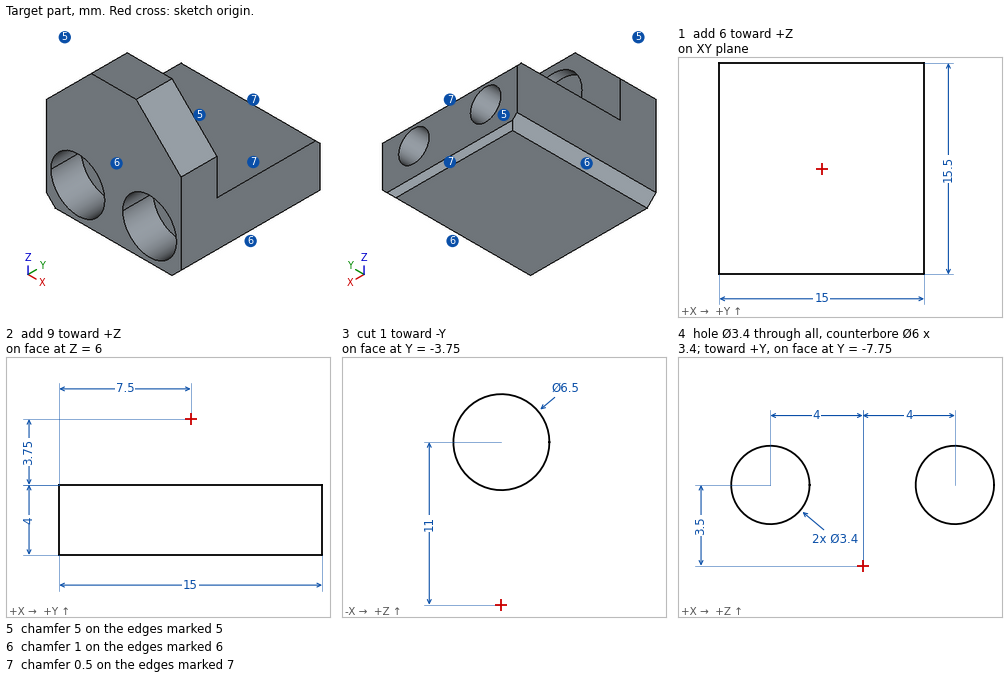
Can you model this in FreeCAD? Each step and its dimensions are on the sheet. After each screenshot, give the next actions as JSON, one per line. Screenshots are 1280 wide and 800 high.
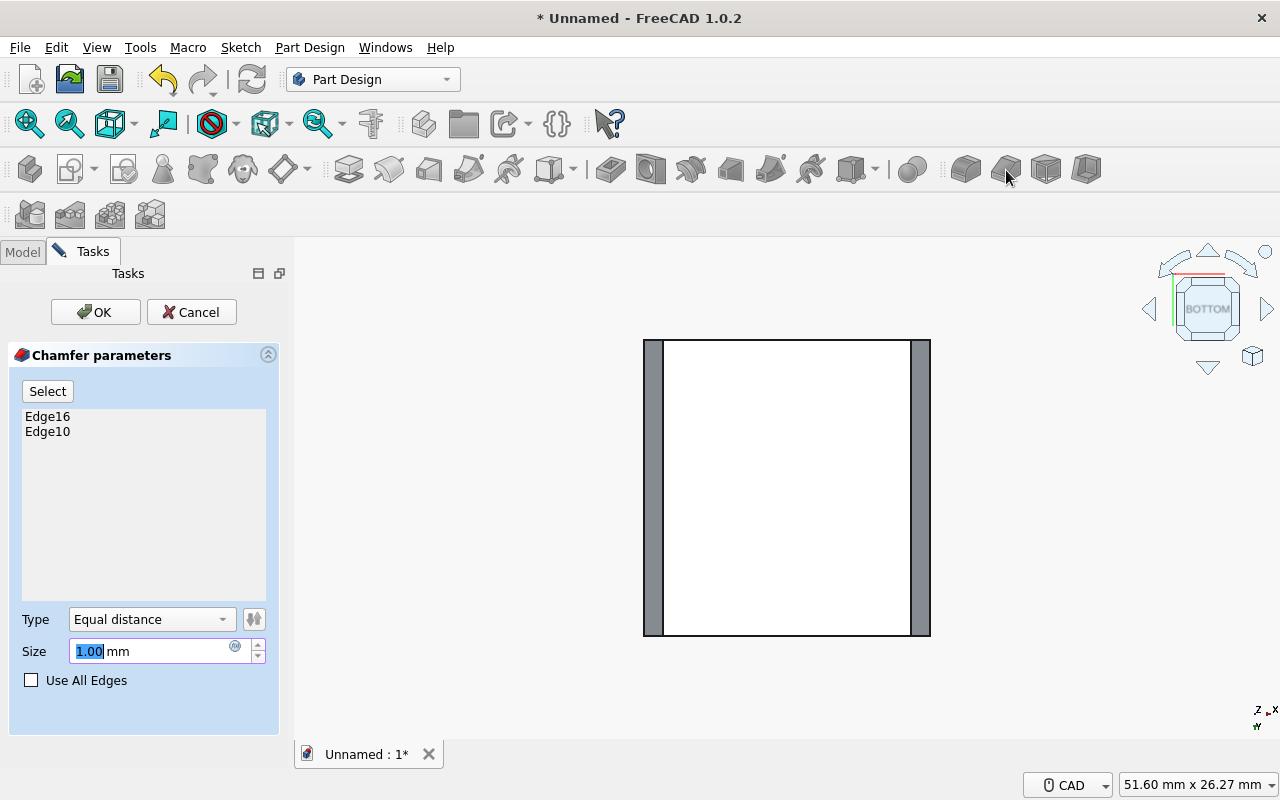
{"action": "type", "text": "1"}
{"action": "key", "text": "Tab"}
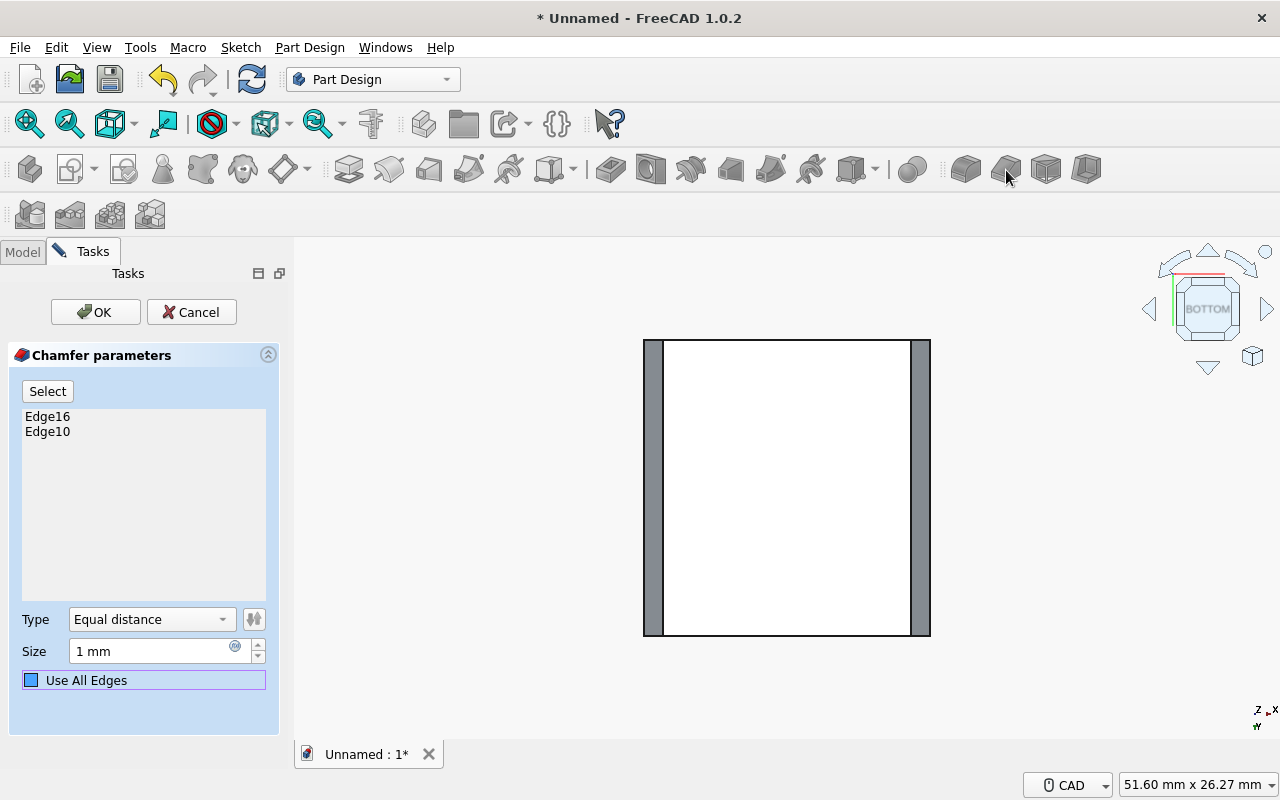
{"action": "left_click", "coordinate": [96, 312]}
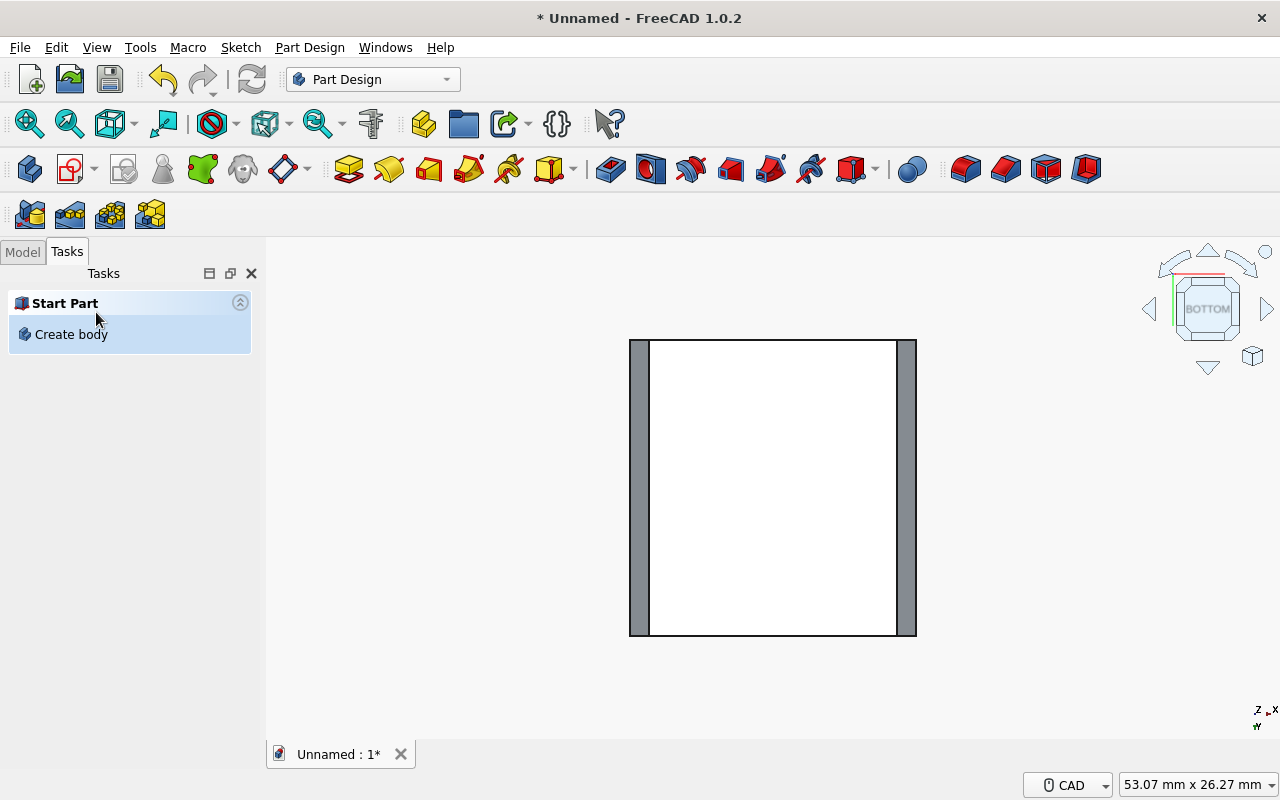
{"action": "left_click", "coordinate": [773, 635]}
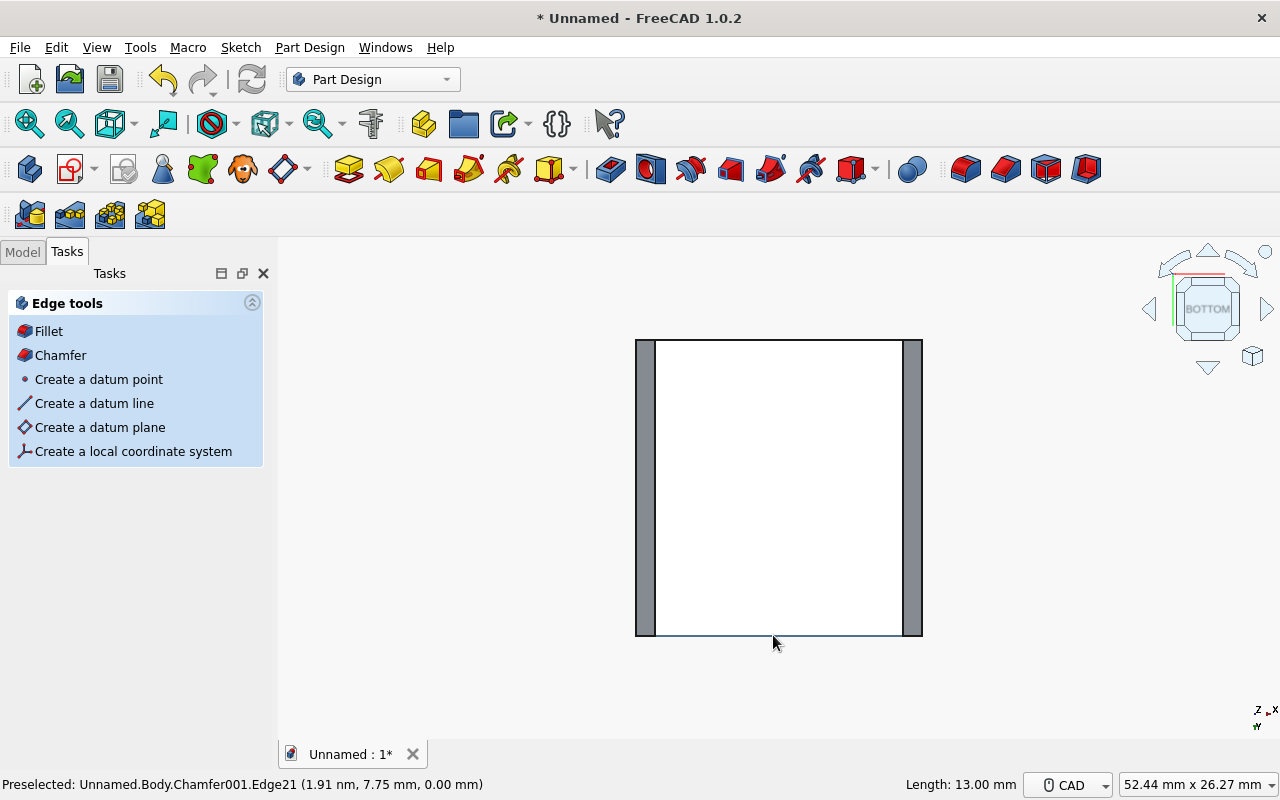
{"action": "key", "text": "0"}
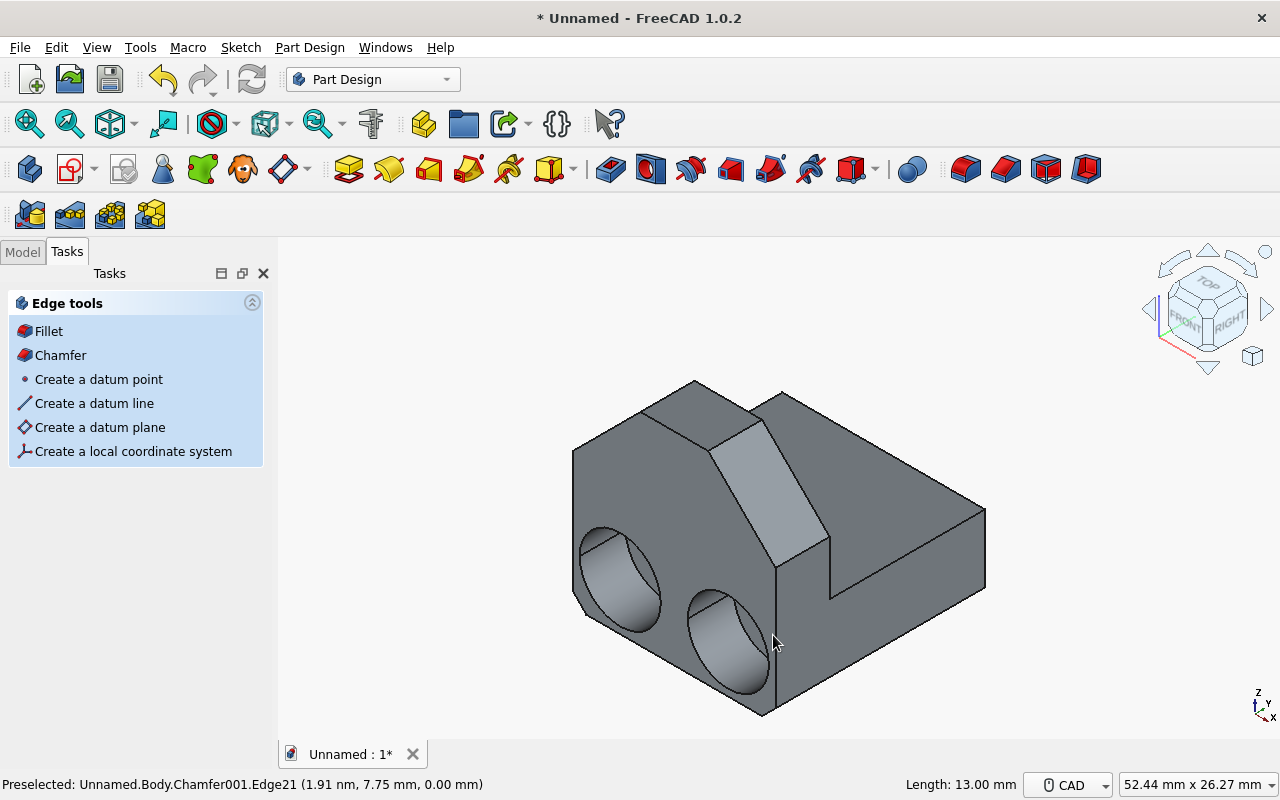
{"action": "key", "text": "2"}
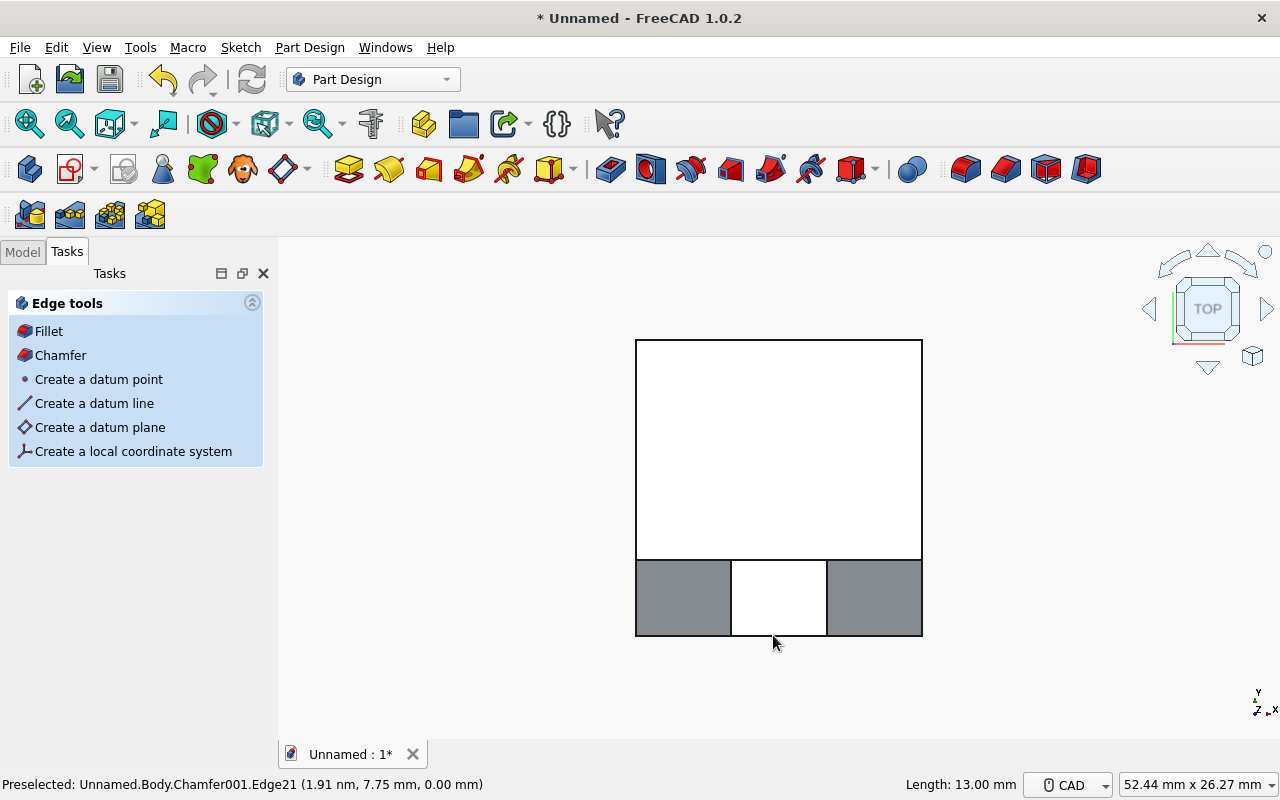
{"action": "left_click", "coordinate": [779, 339], "text": "ctrl"}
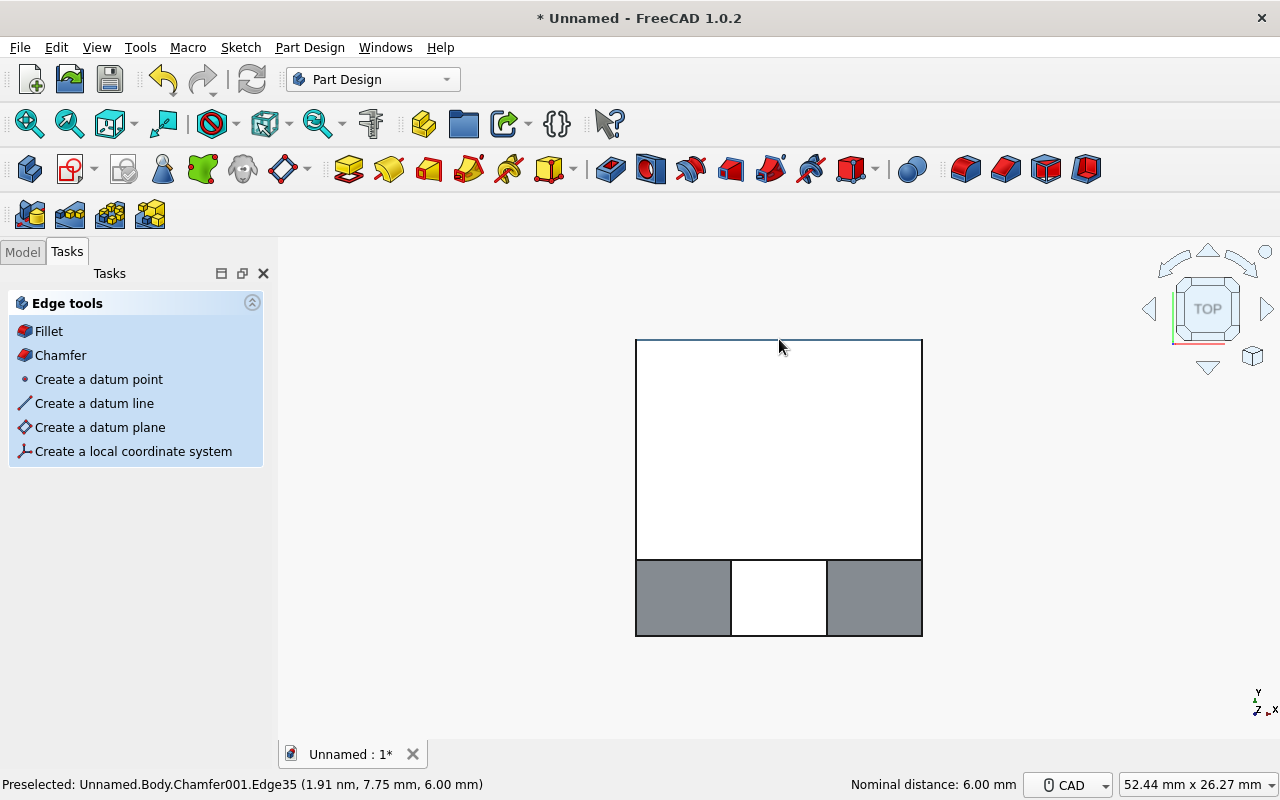
{"action": "left_click", "coordinate": [1006, 170]}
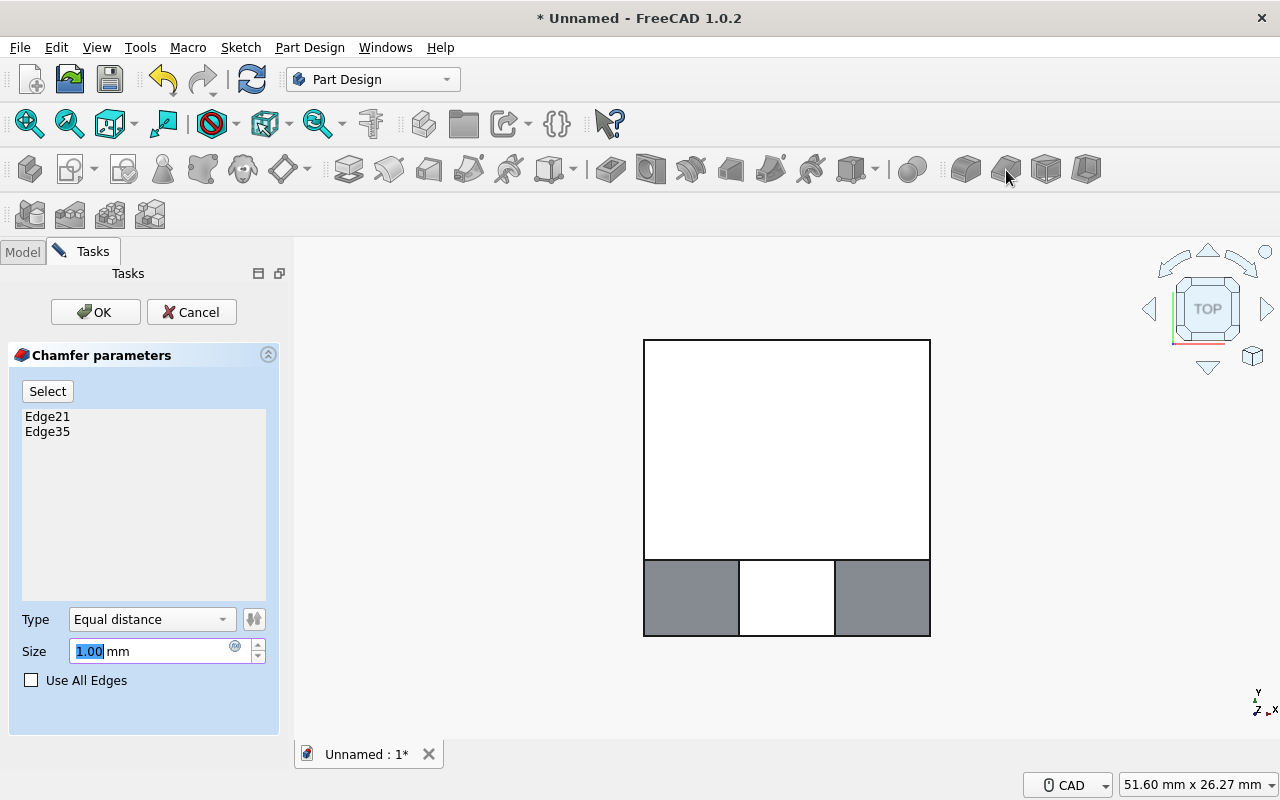
{"action": "type", "text": "0.5"}
{"action": "key", "text": "Tab"}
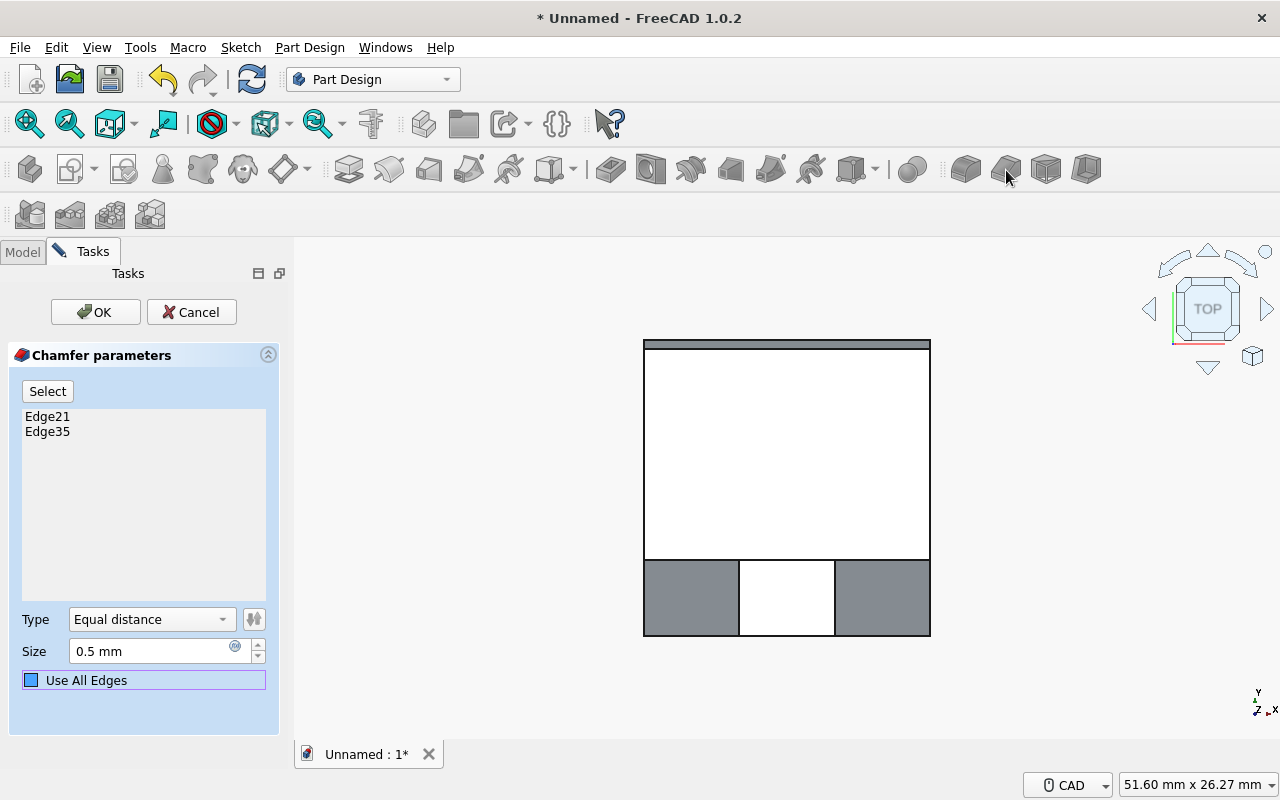
{"action": "left_click", "coordinate": [96, 312]}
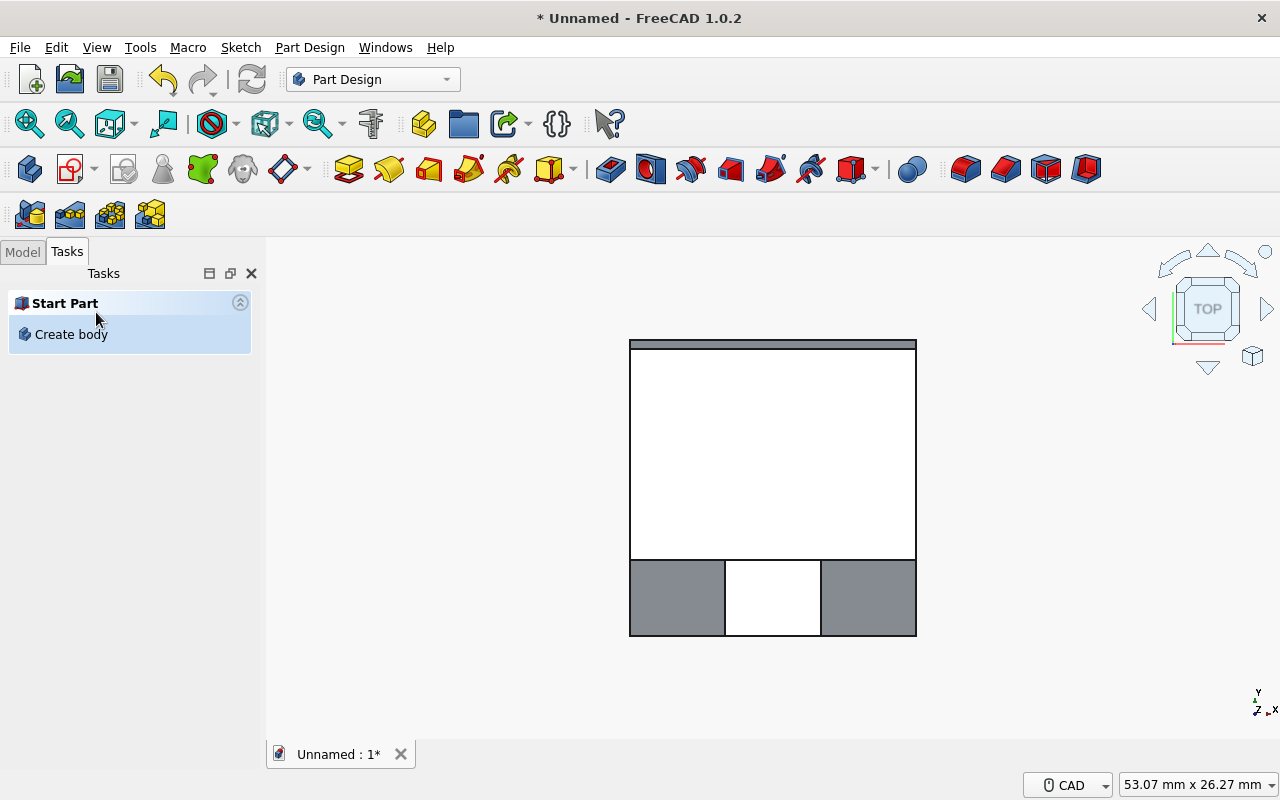
{"action": "key", "text": "0"}